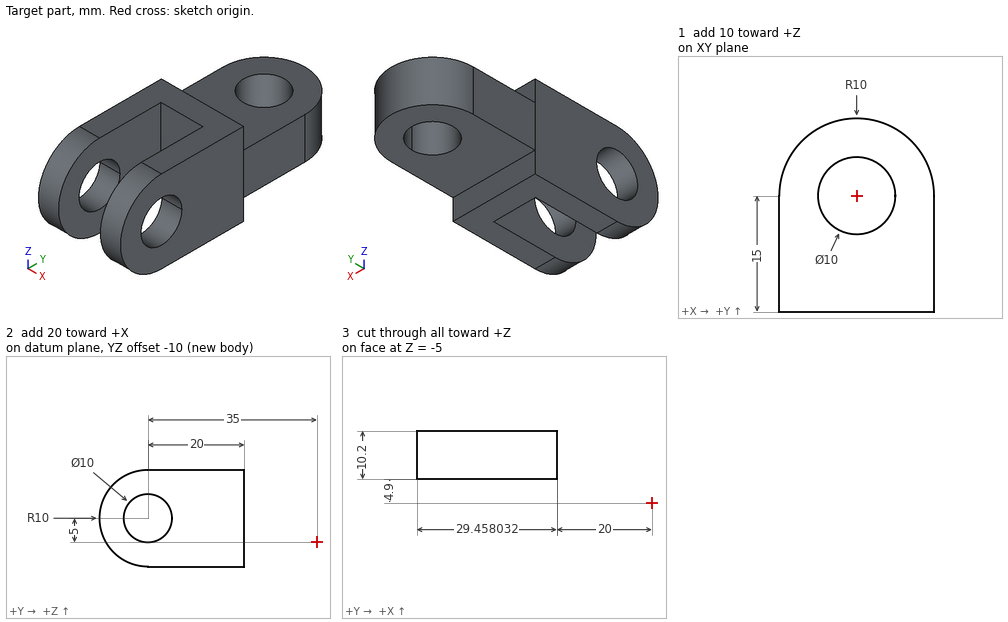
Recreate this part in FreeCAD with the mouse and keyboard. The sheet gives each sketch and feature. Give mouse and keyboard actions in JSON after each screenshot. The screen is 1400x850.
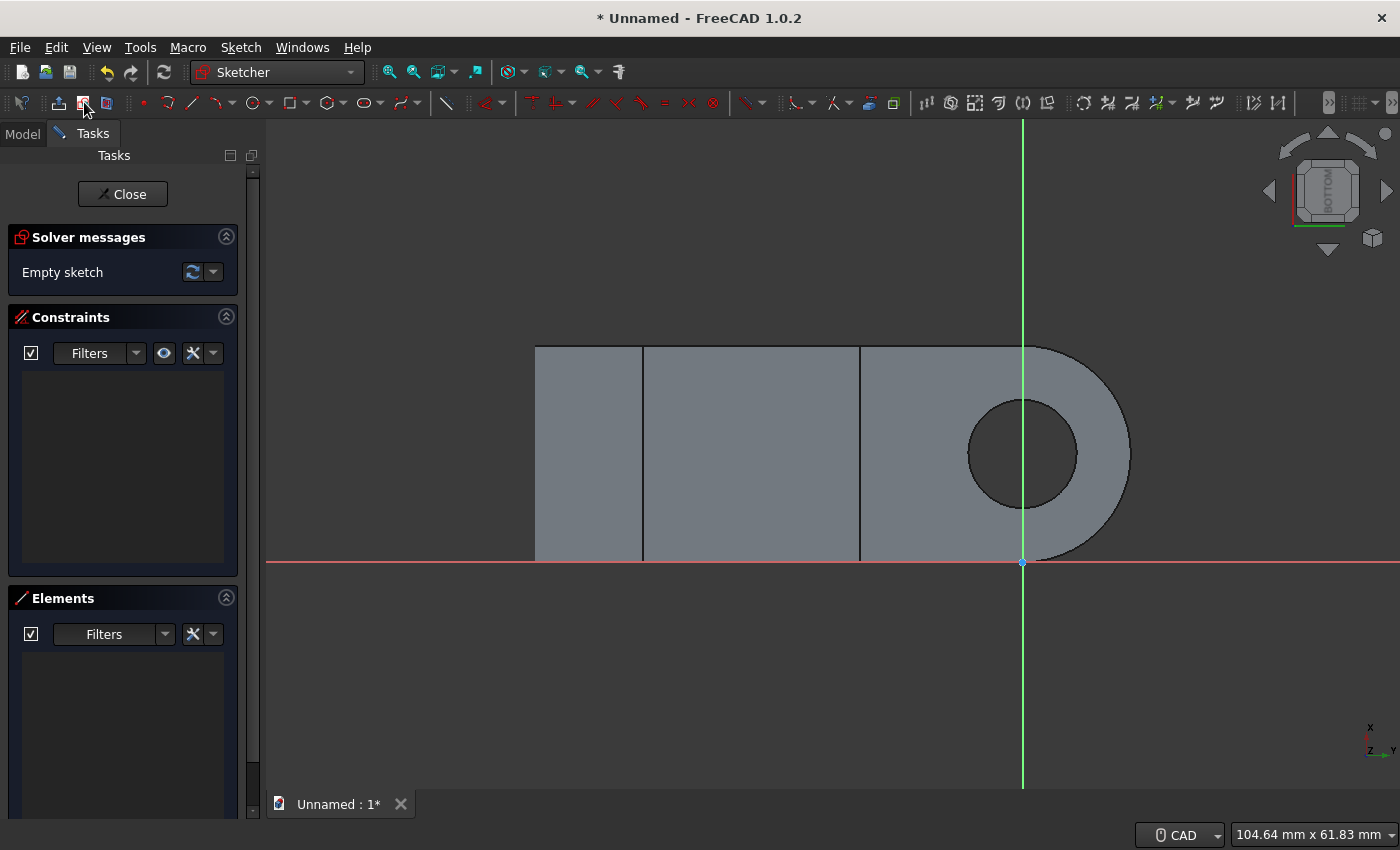
{"action": "left_click", "coordinate": [290, 104]}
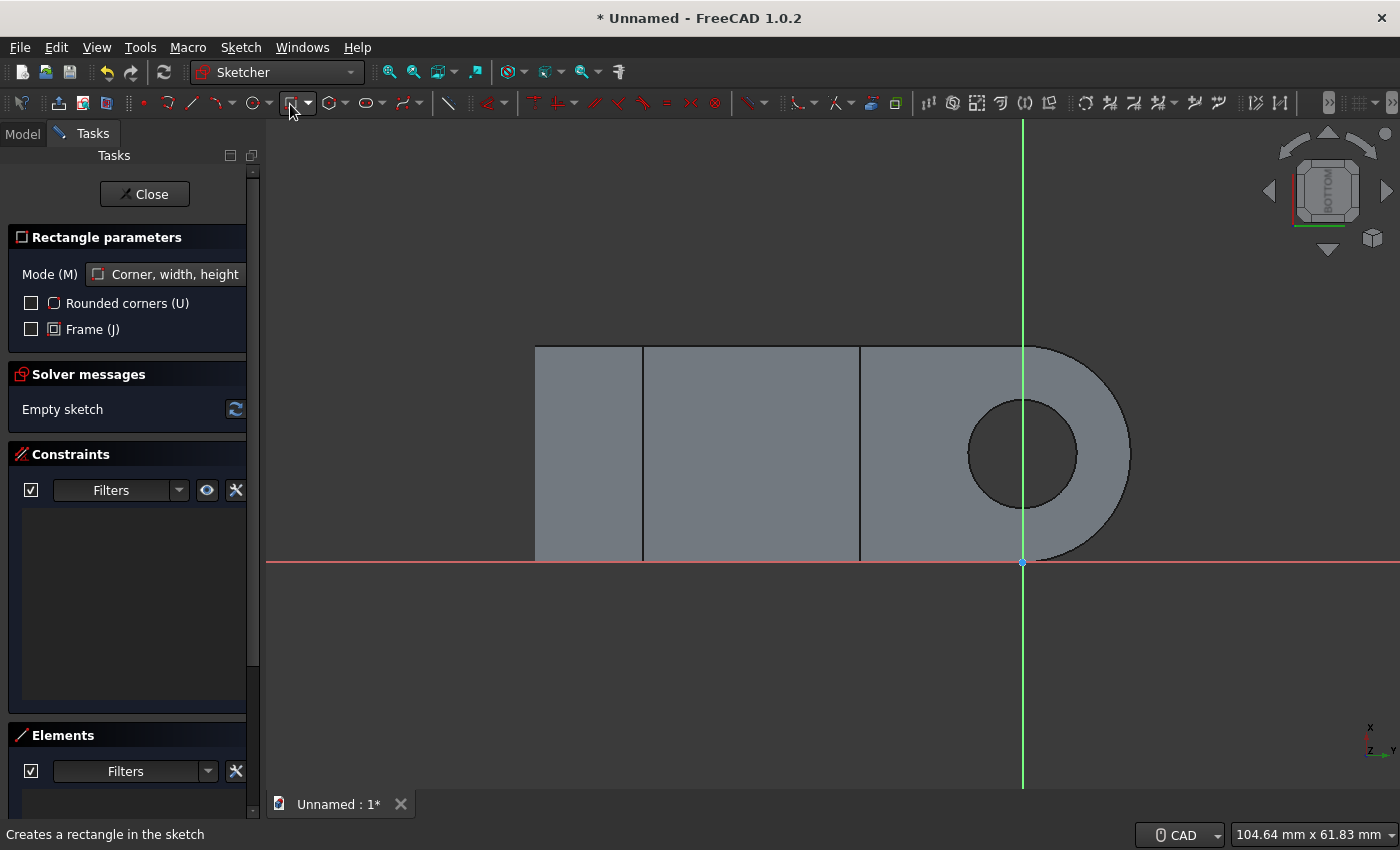
{"action": "left_click", "coordinate": [487, 399]}
{"action": "left_click", "coordinate": [806, 509]}
{"action": "key", "text": "Escape"}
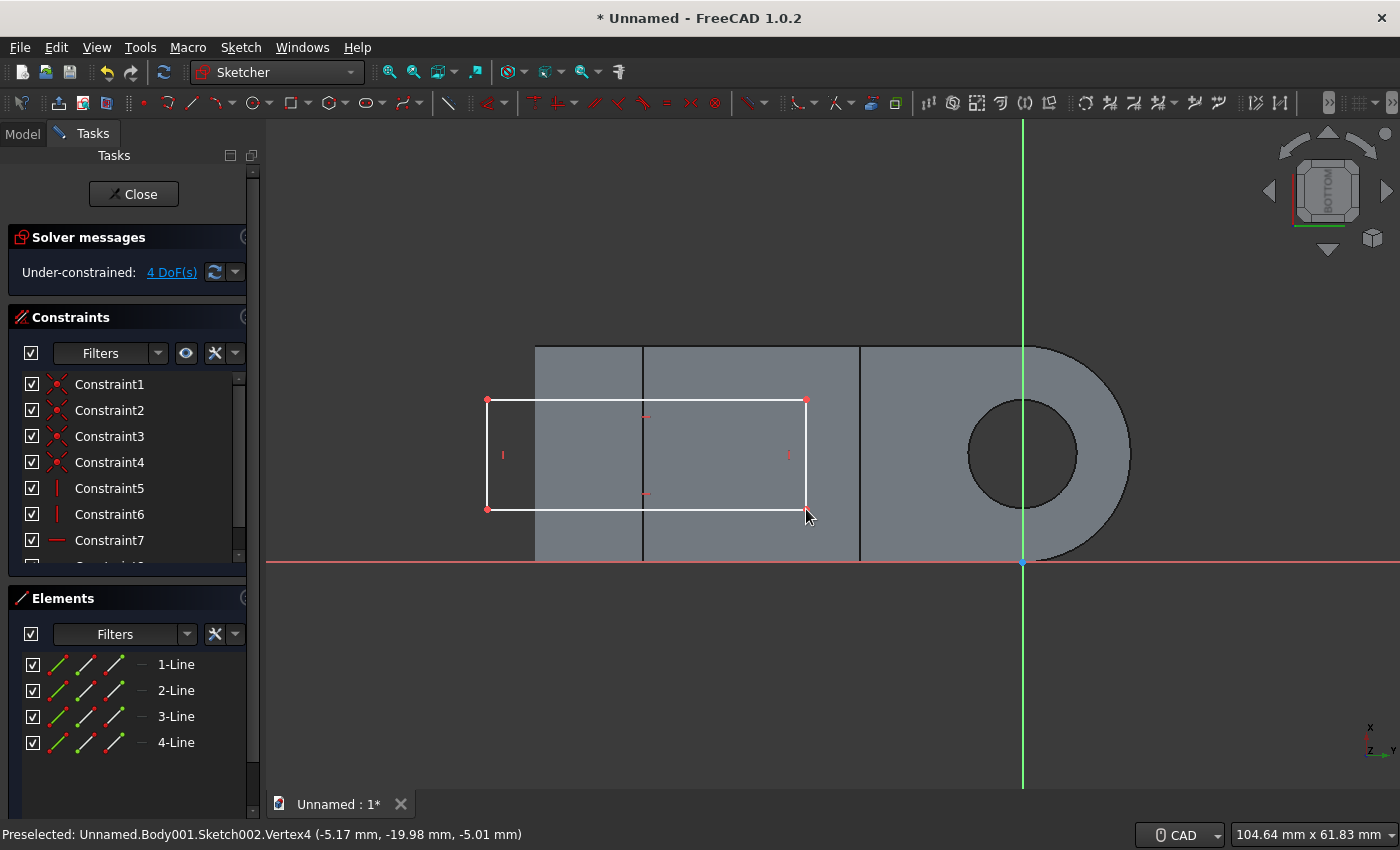
{"action": "left_click", "coordinate": [488, 104]}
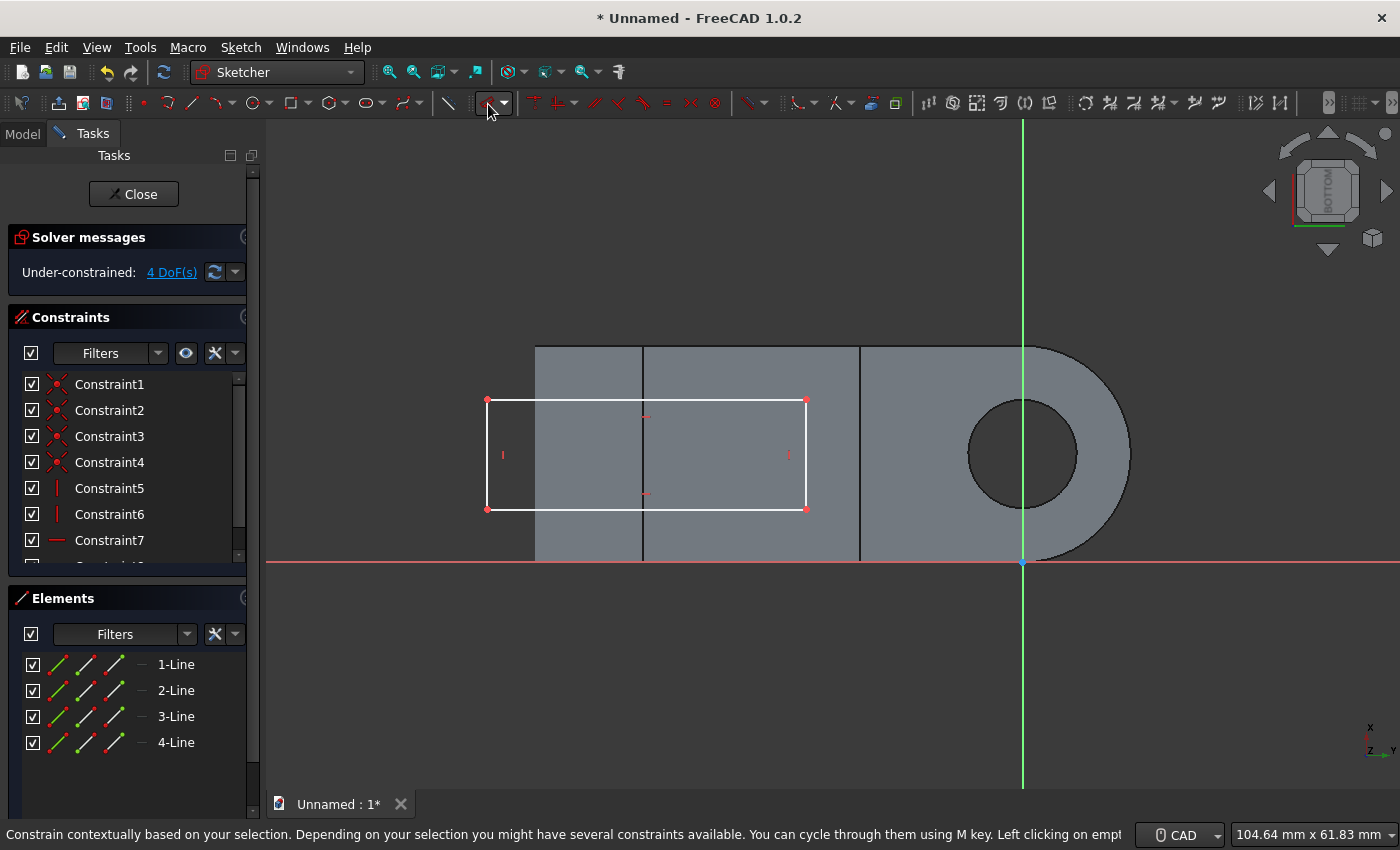
{"action": "left_click", "coordinate": [806, 510]}
{"action": "left_click", "coordinate": [914, 596]}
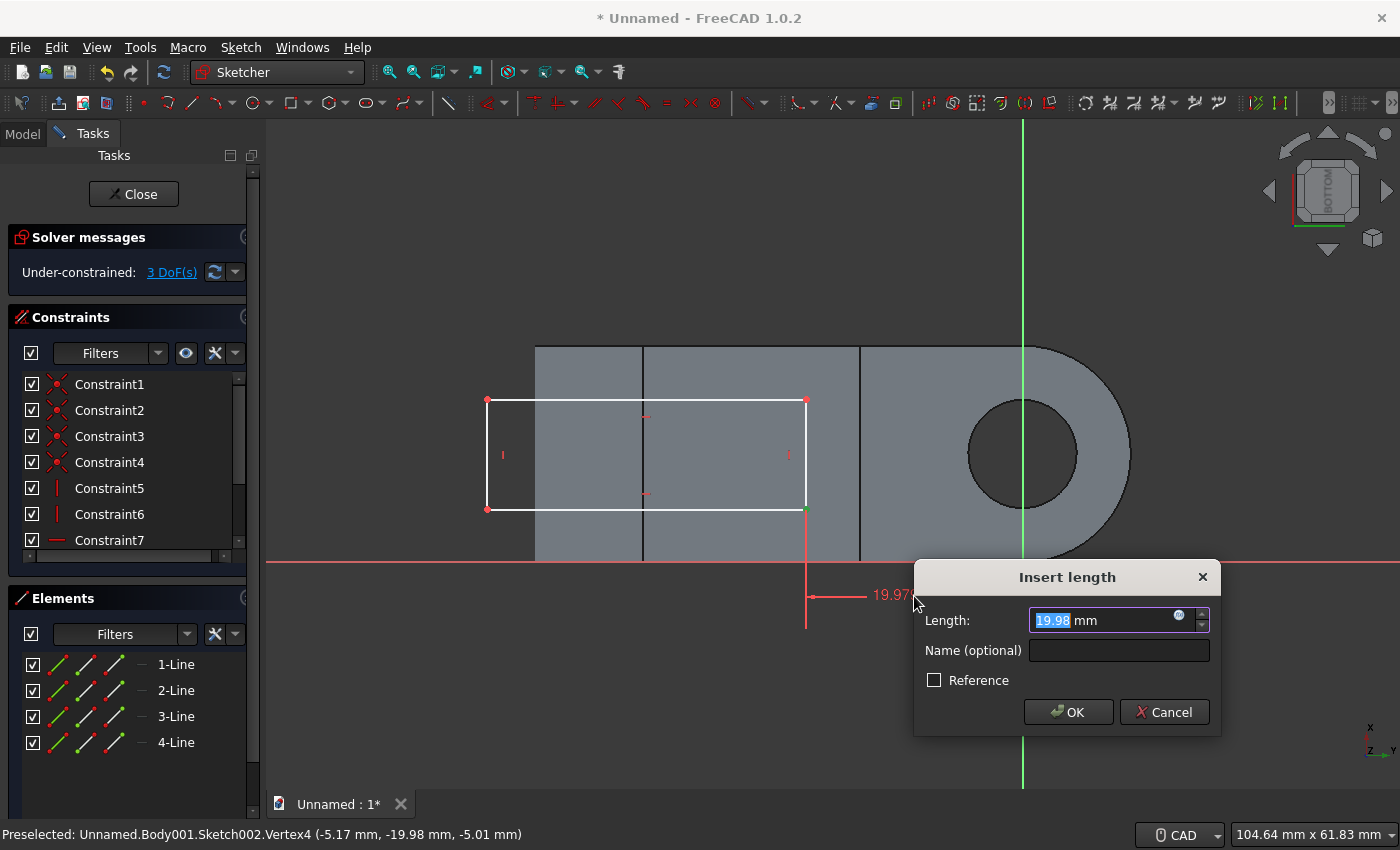
{"action": "type", "text": "20"}
{"action": "key", "text": "Return"}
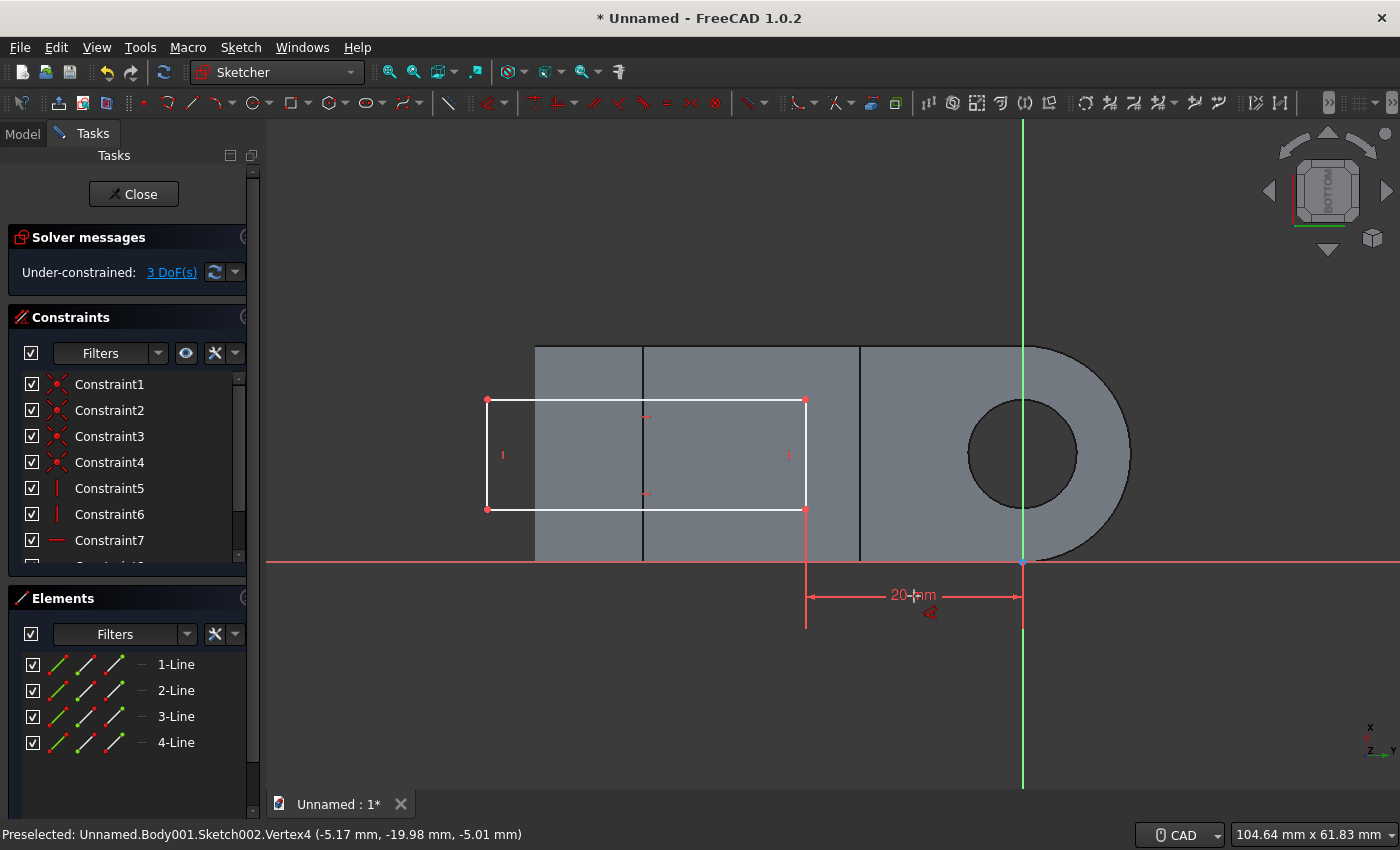
{"action": "left_click", "coordinate": [487, 433]}
{"action": "left_click", "coordinate": [453, 455]}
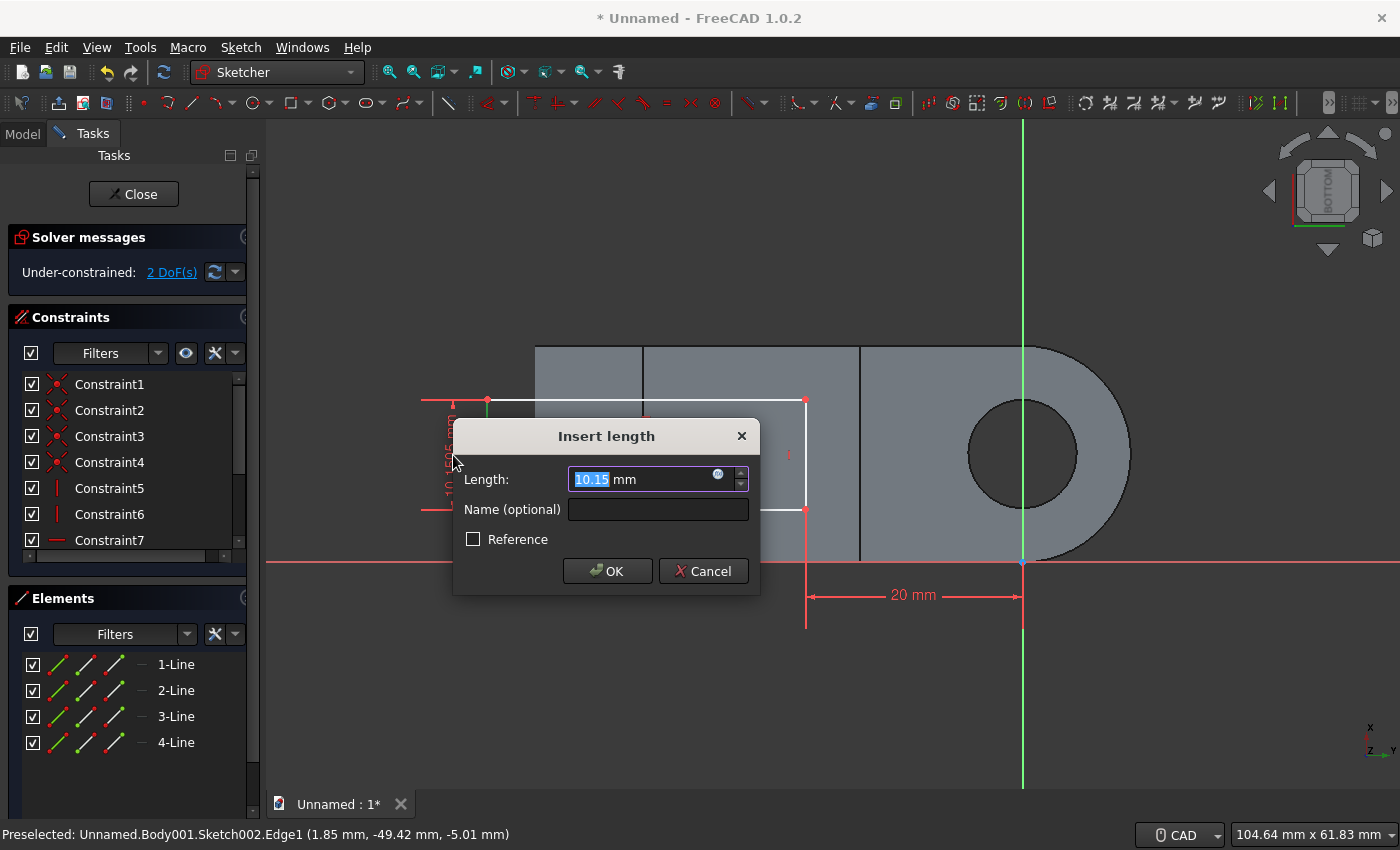
{"action": "type", "text": "10.2"}
{"action": "key", "text": "Return"}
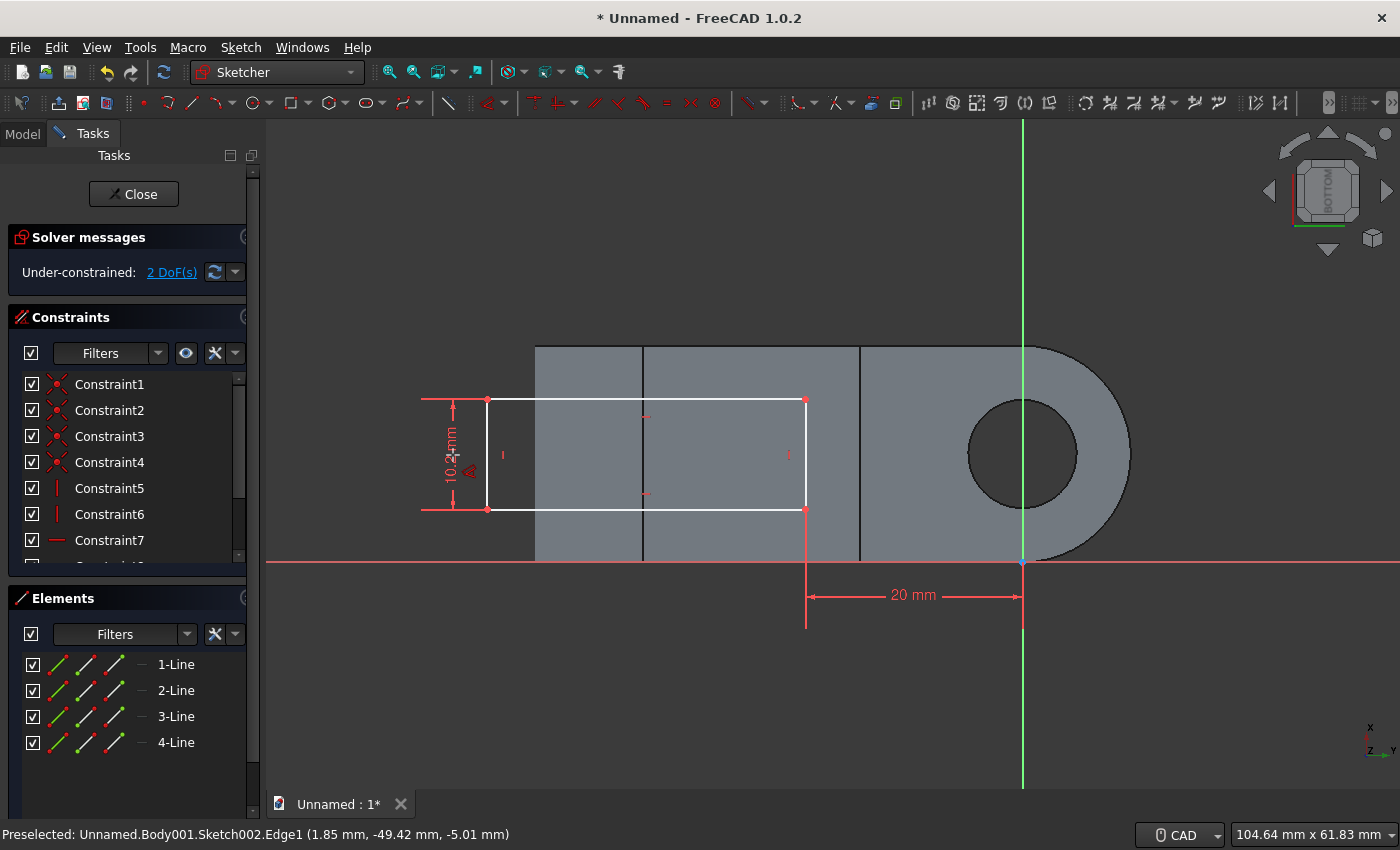
{"action": "left_click", "coordinate": [487, 510]}
{"action": "left_click", "coordinate": [1057, 536]}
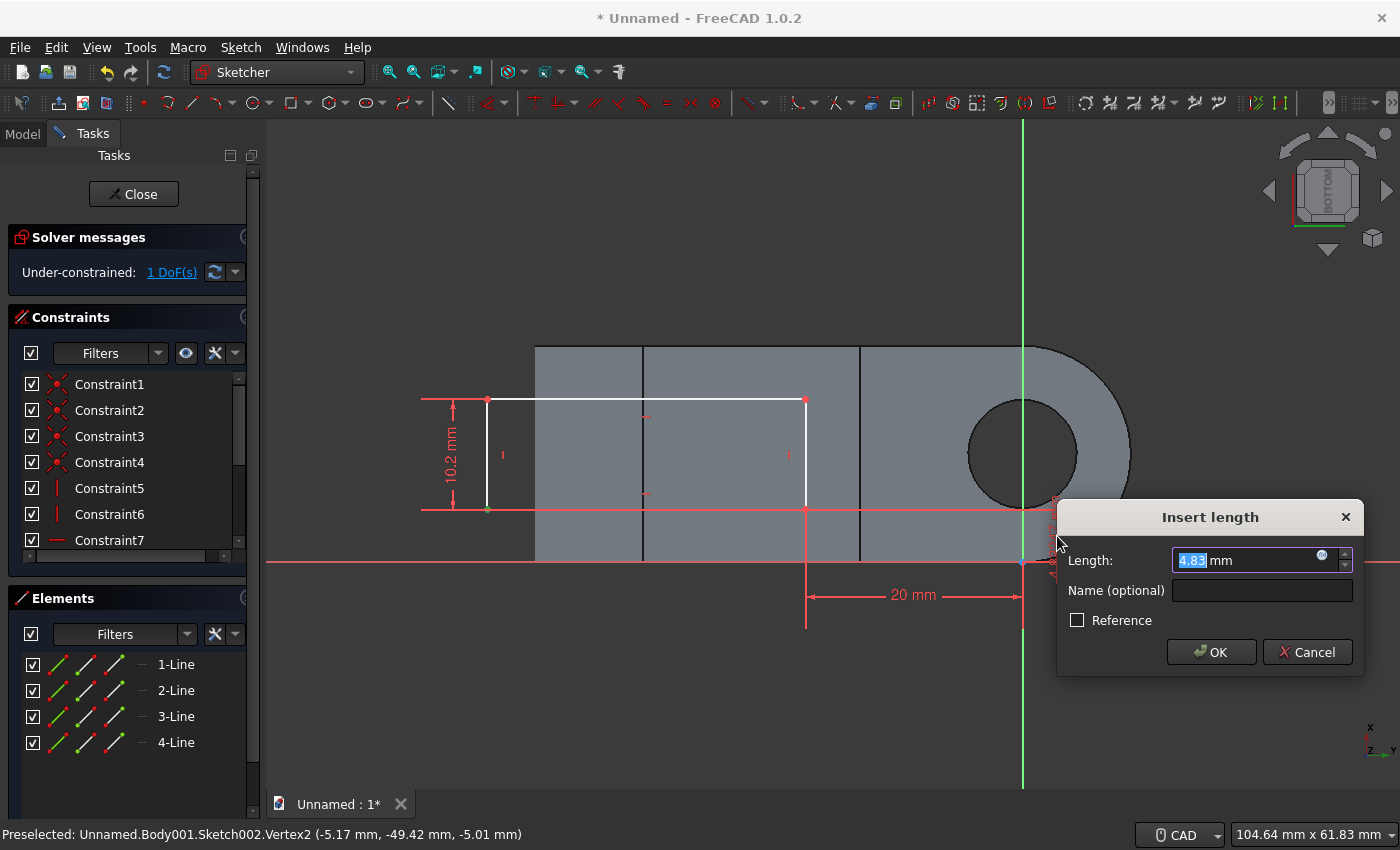
{"action": "type", "text": "4.9"}
{"action": "key", "text": "Return"}